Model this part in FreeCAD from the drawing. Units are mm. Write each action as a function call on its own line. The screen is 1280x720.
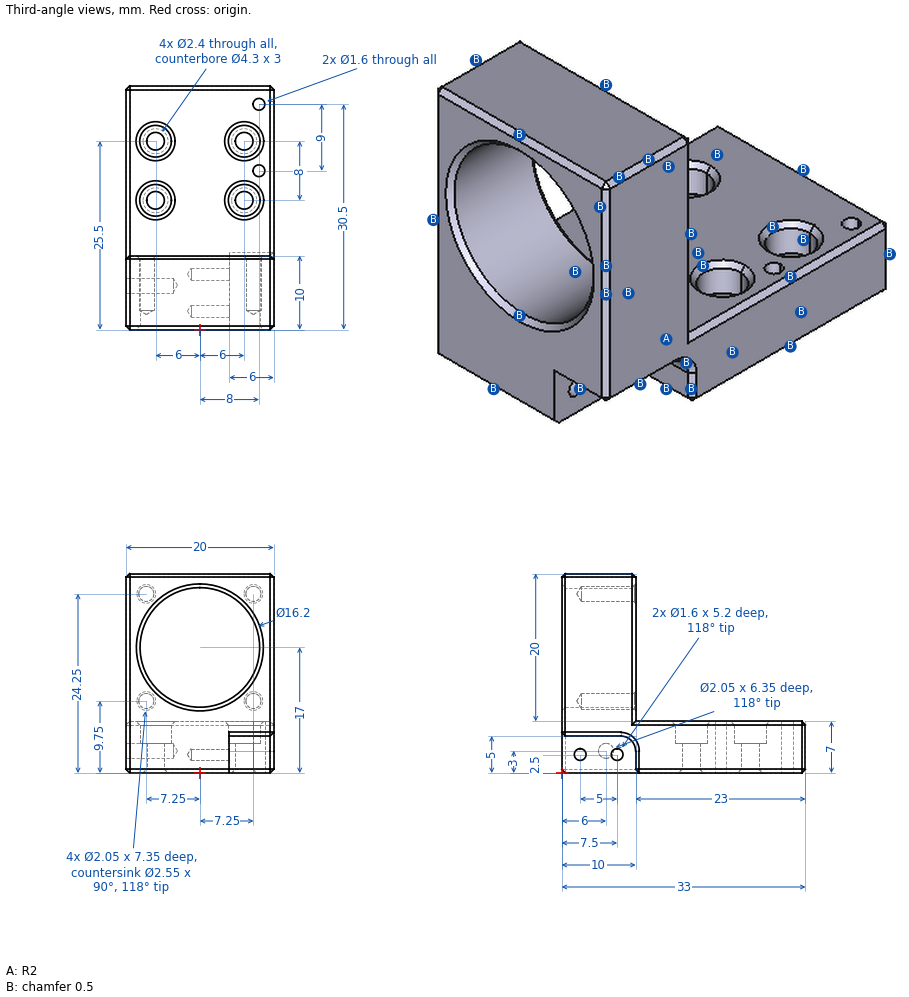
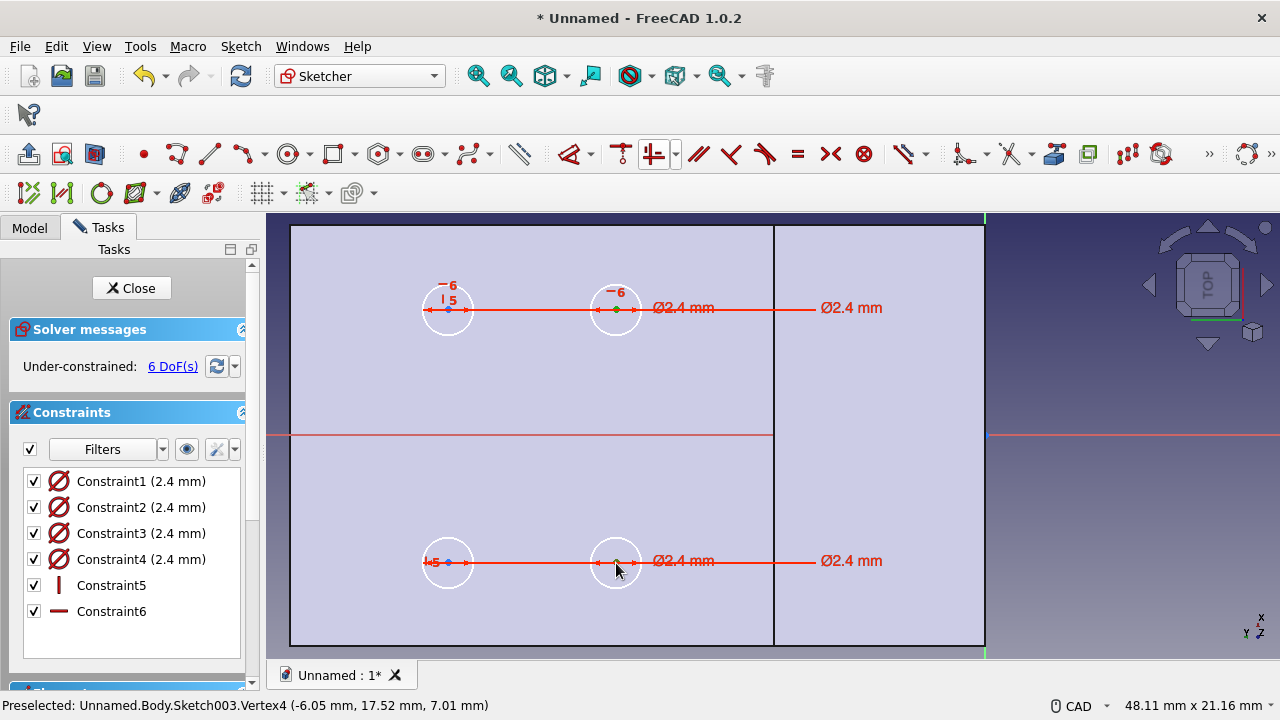
key(v)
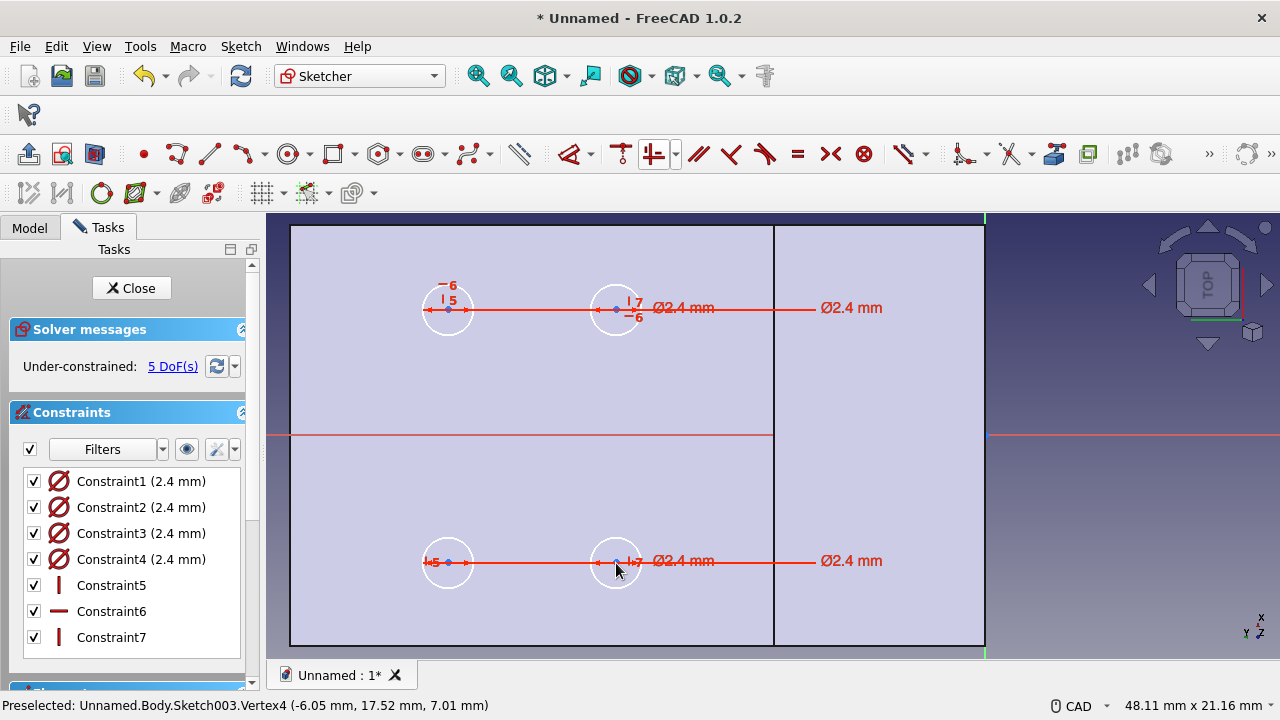
click(448, 563)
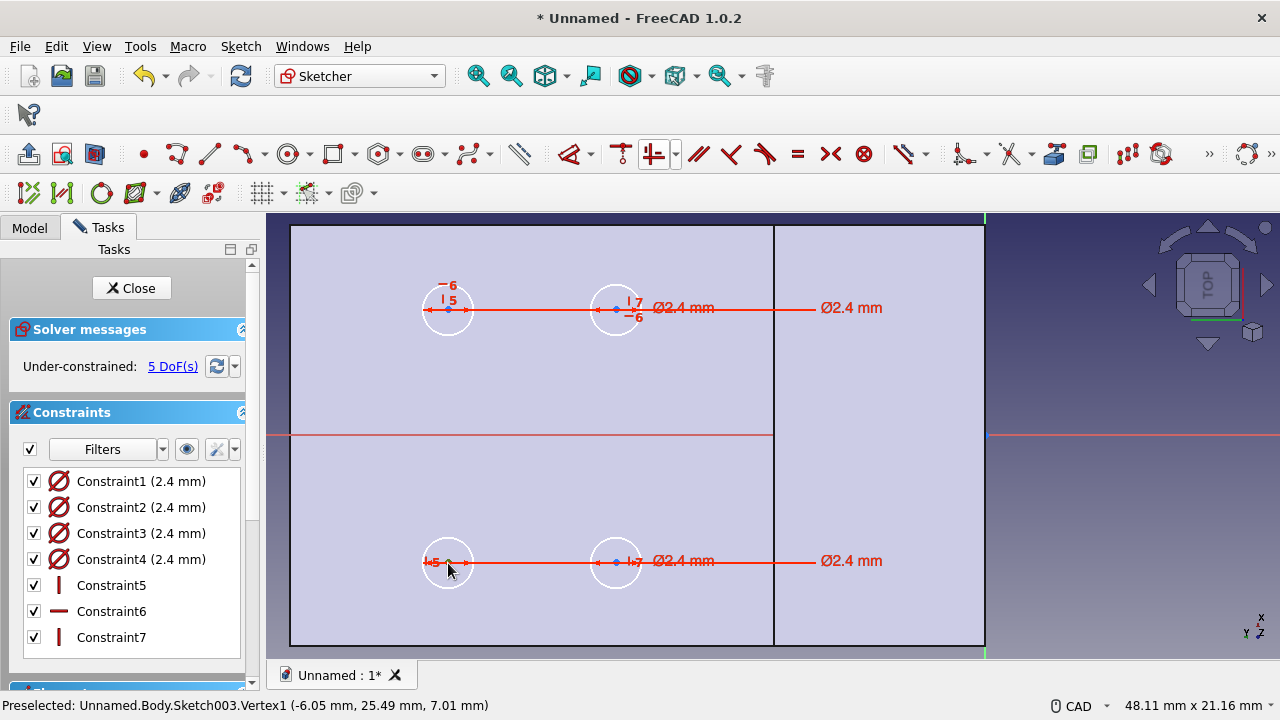
click(616, 563)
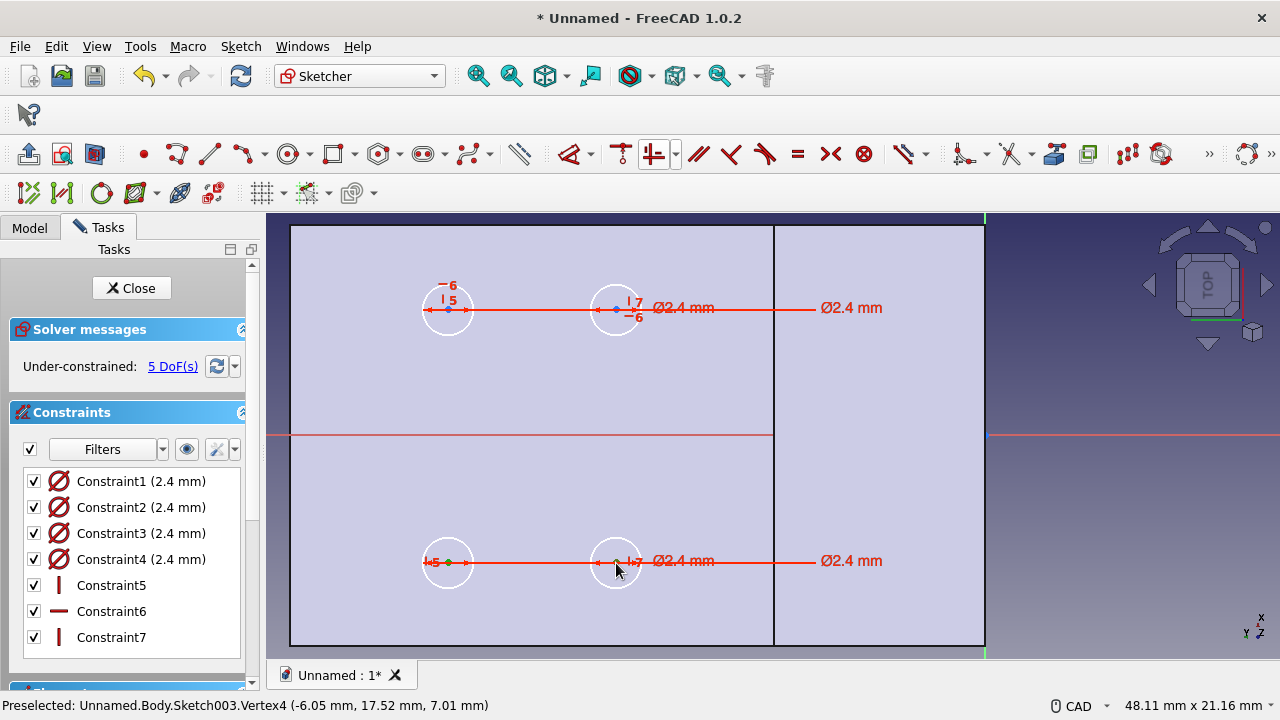
key(h)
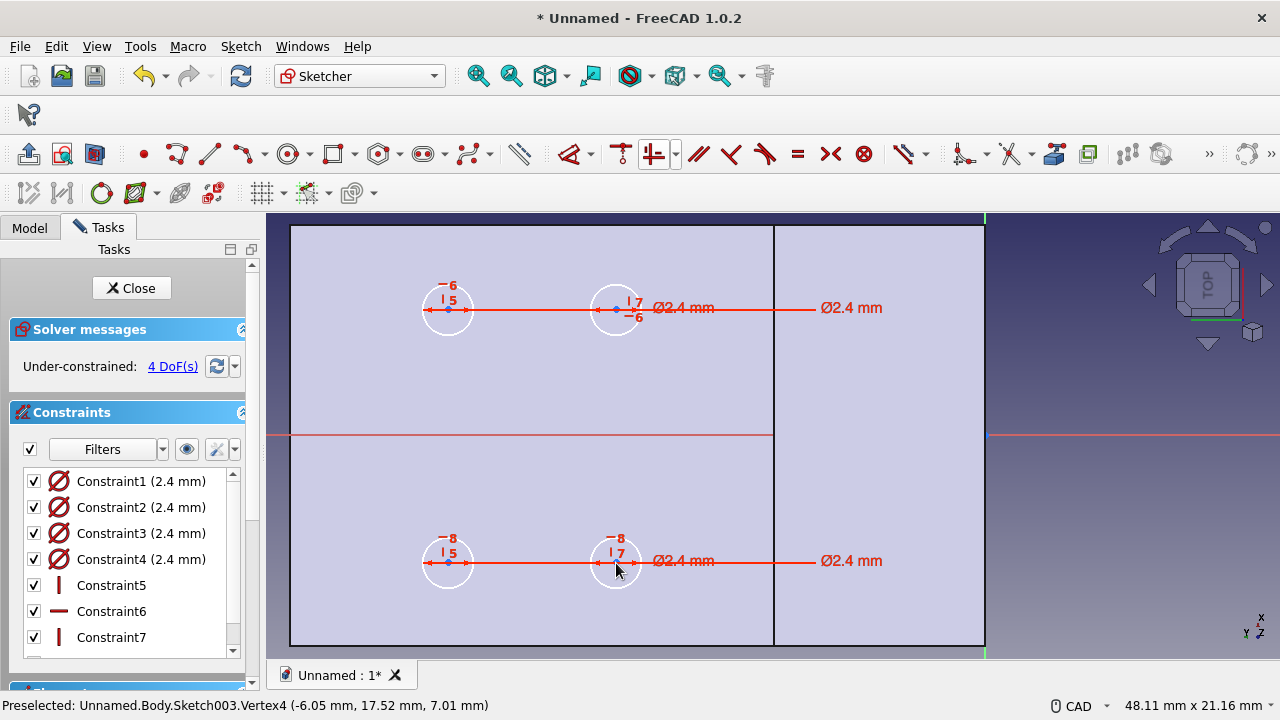
click(568, 154)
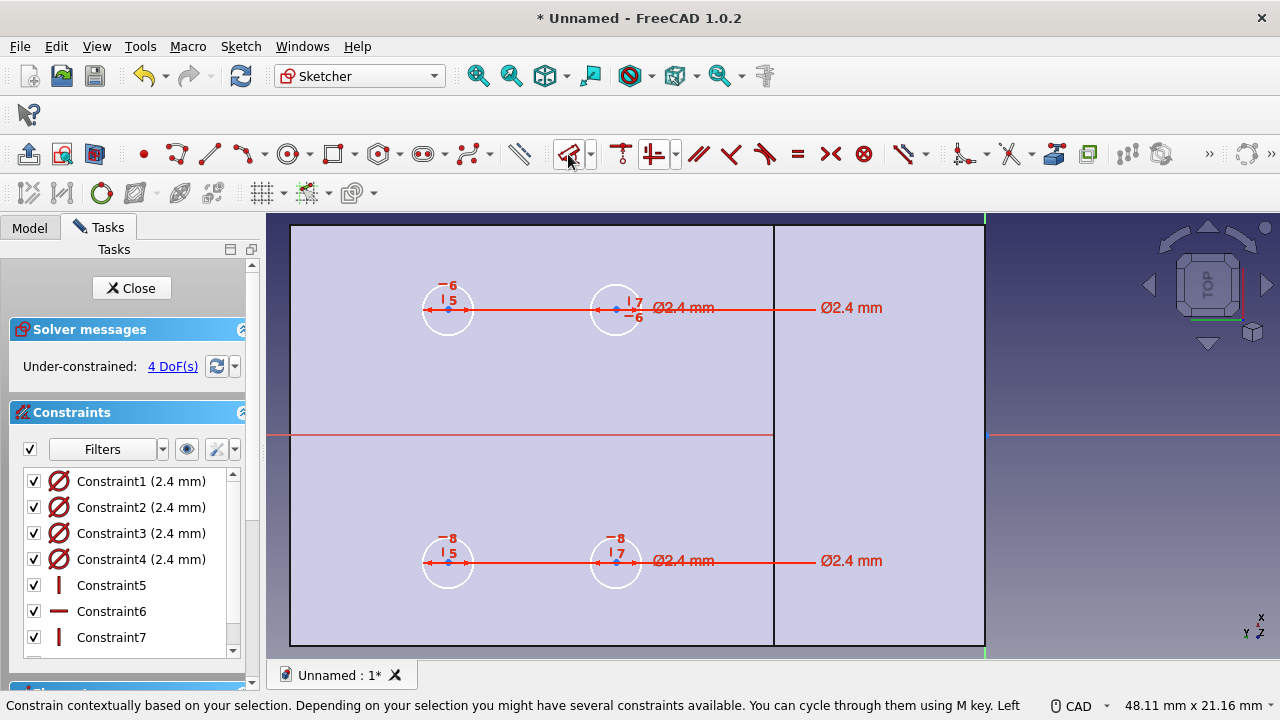
click(448, 563)
click(1019, 499)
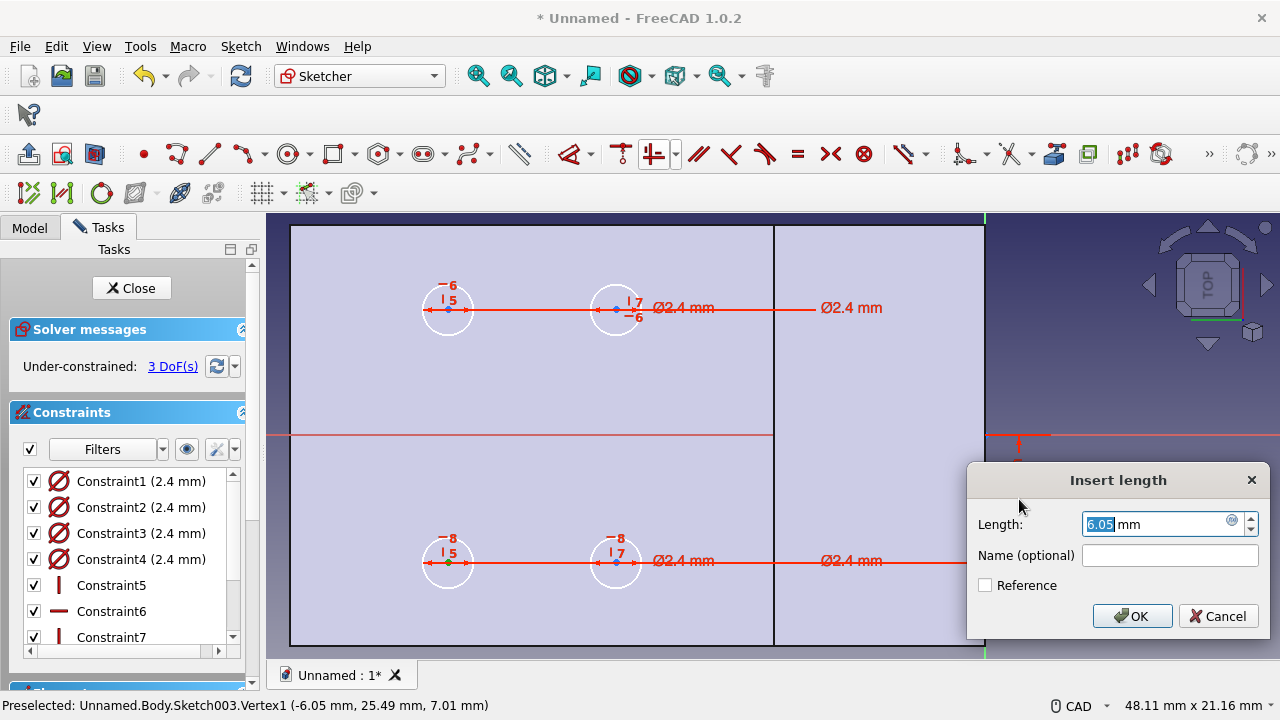
text(6)
key(Return)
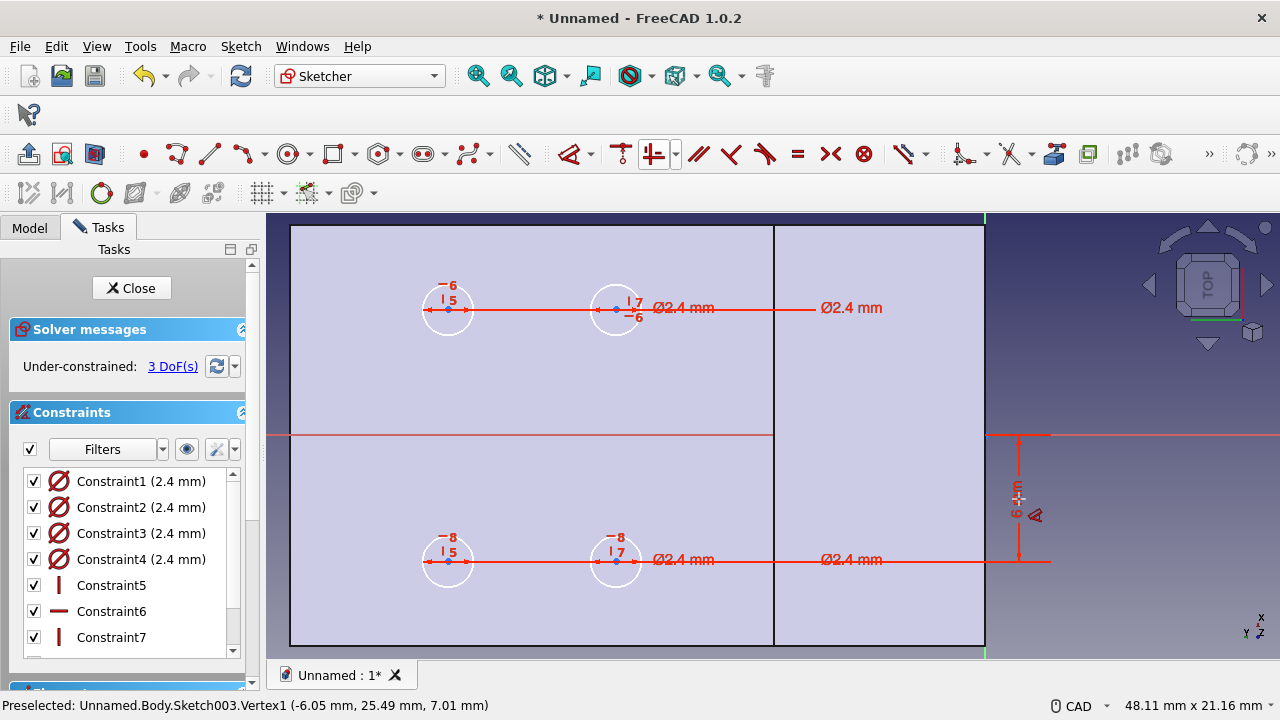
click(448, 310)
click(1019, 373)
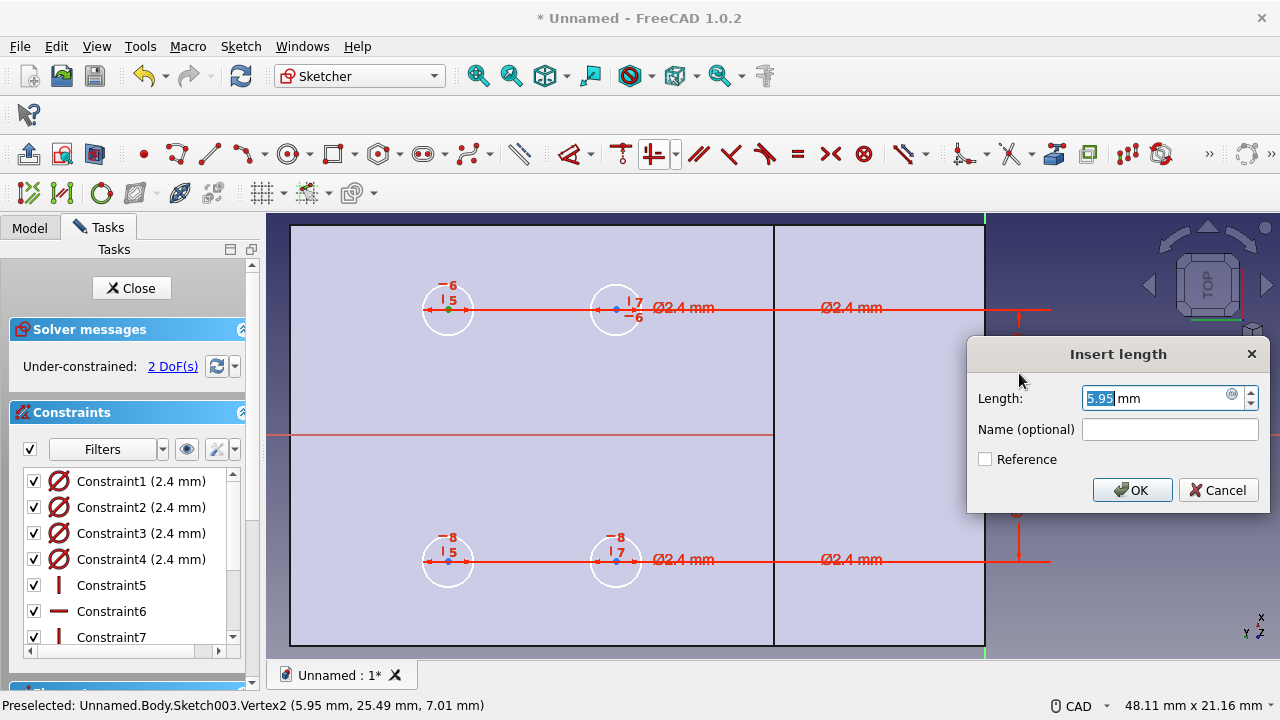
text(6)
key(Return)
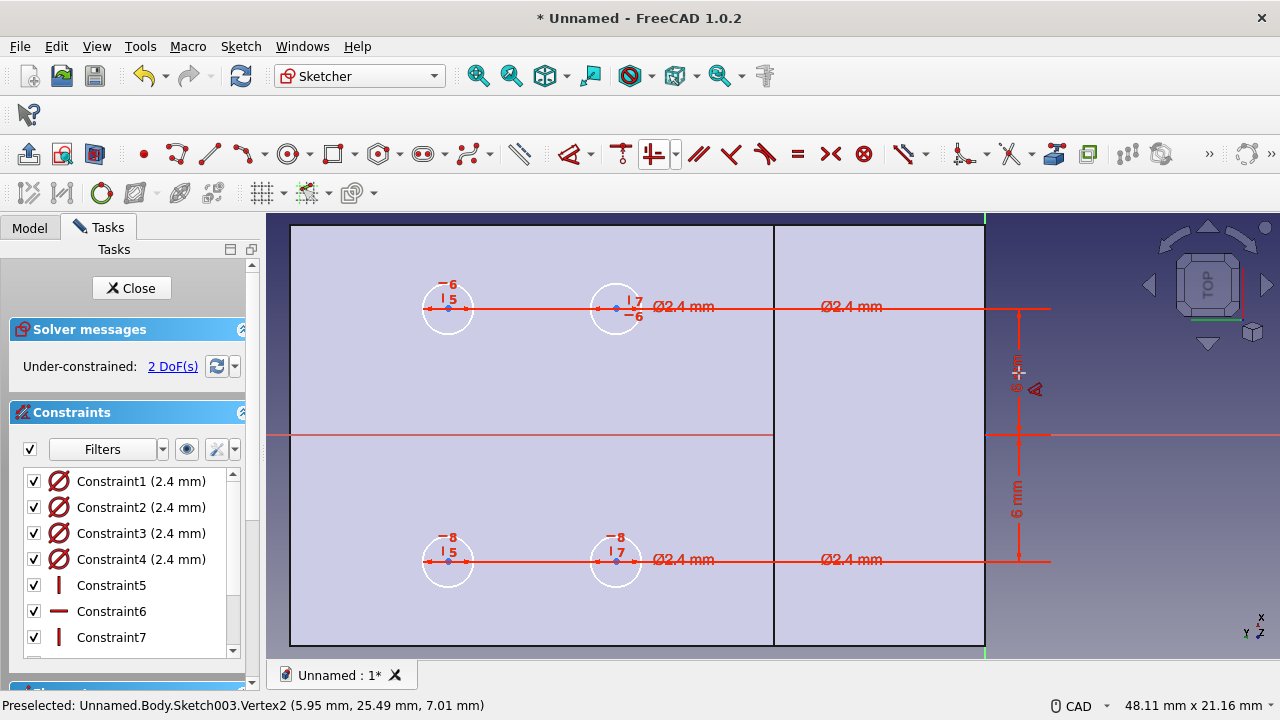
click(448, 309)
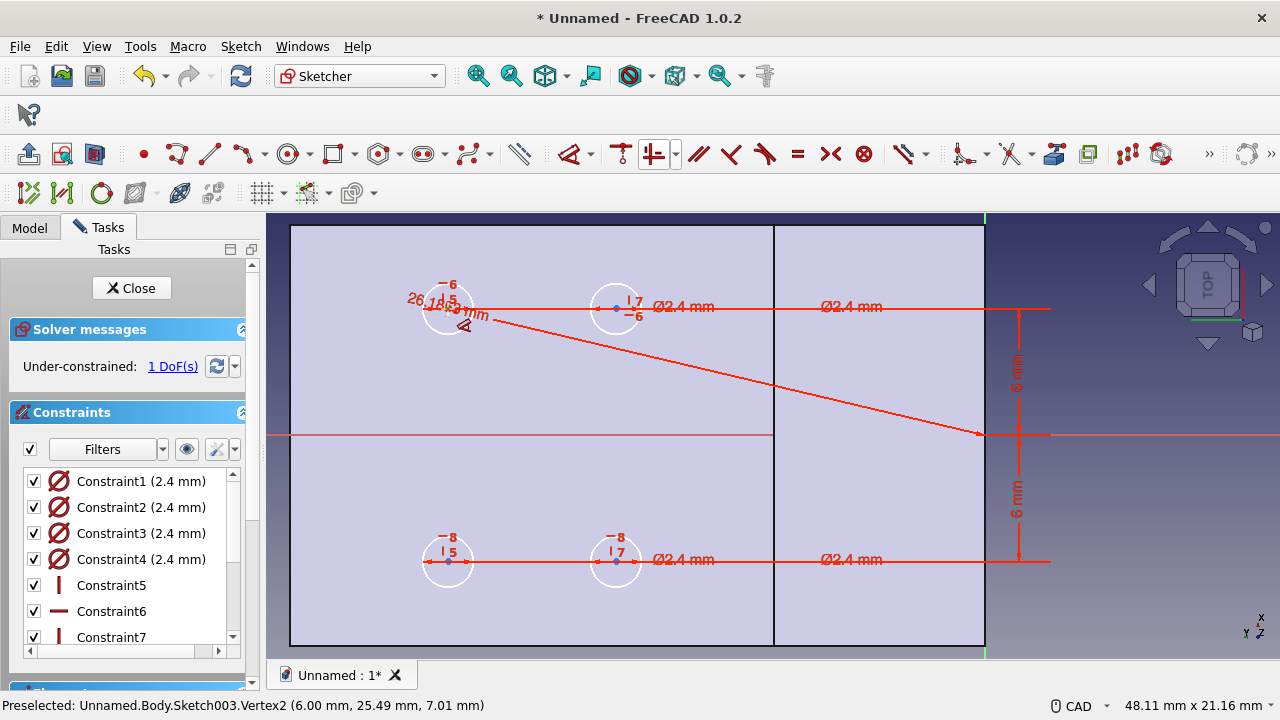
click(616, 309)
click(532, 275)